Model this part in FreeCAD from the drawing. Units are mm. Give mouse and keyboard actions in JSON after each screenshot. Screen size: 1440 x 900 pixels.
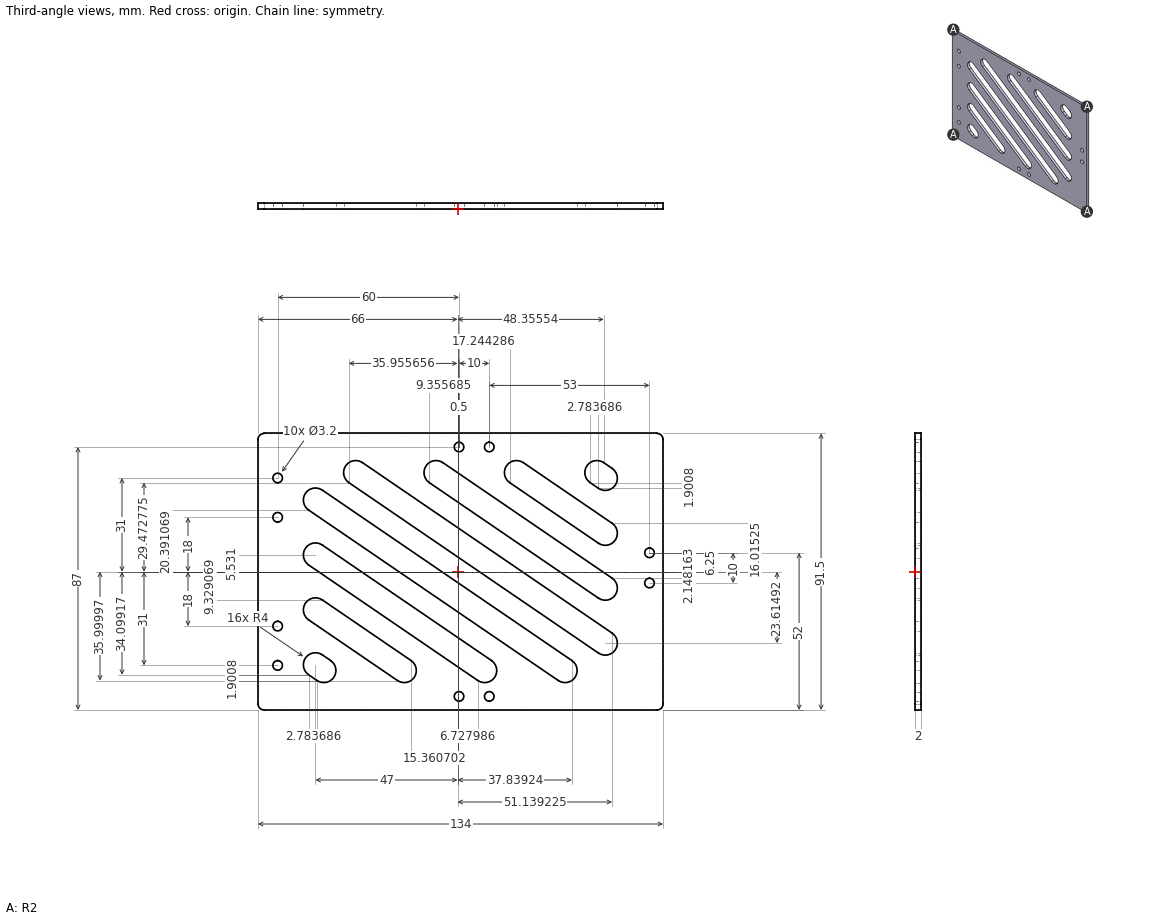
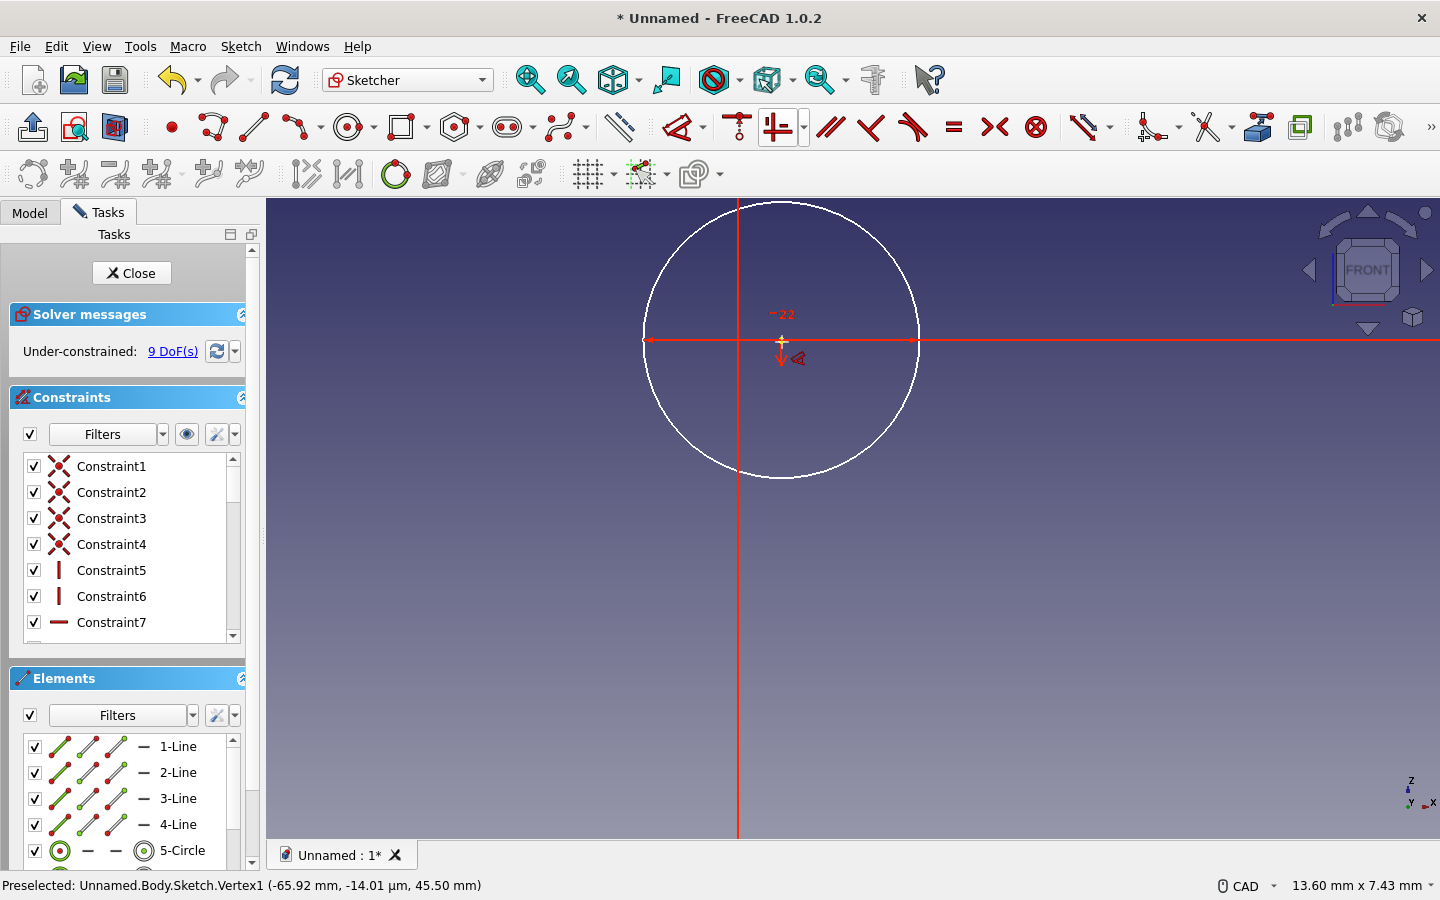
{"action": "left_click", "coordinate": [781, 340]}
{"action": "left_click", "coordinate": [760, 306]}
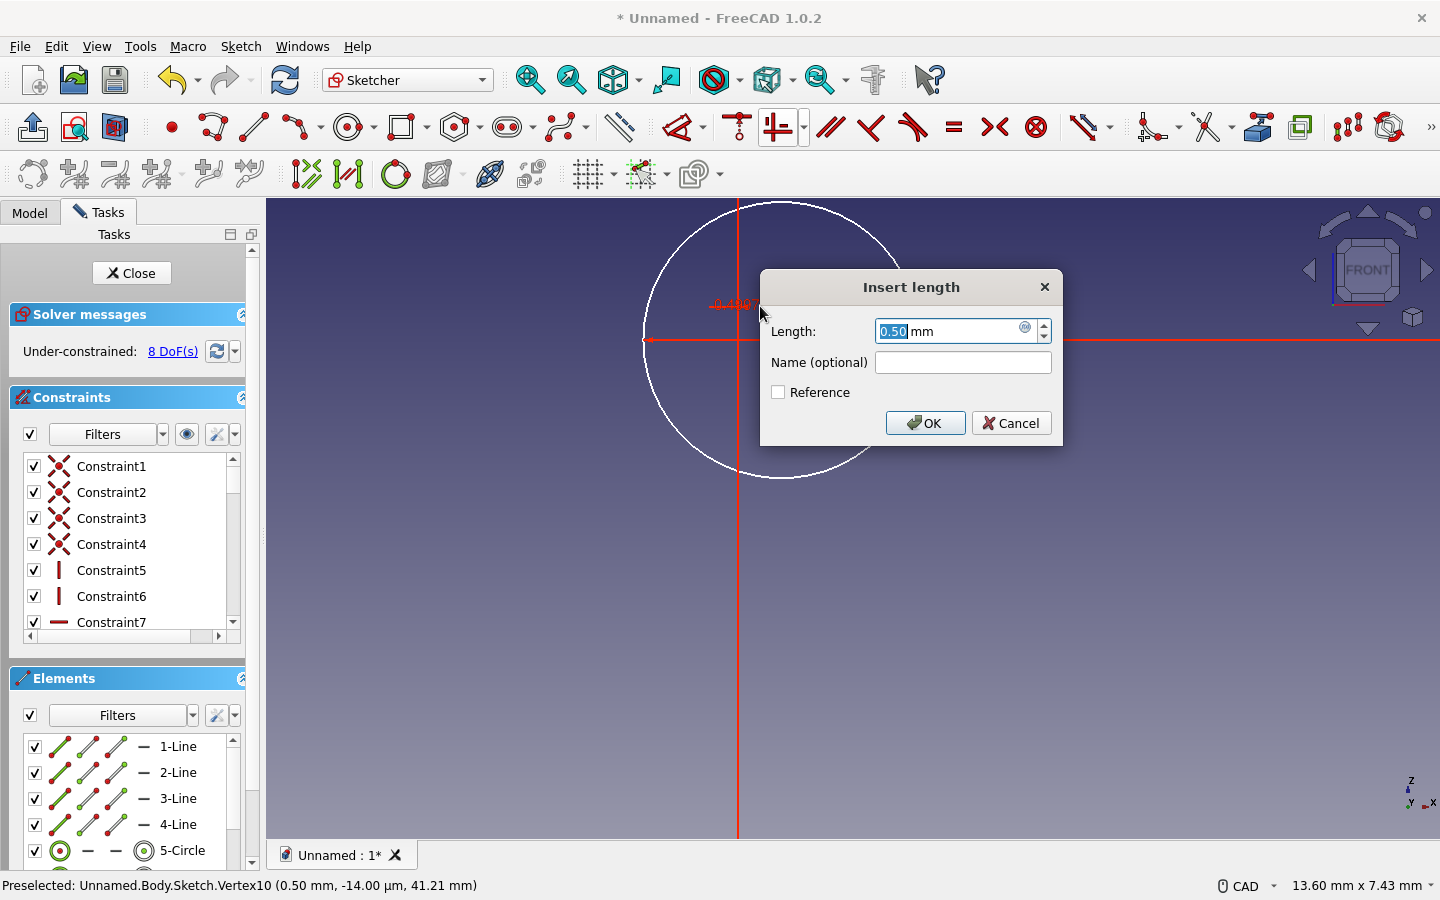
{"action": "type", "text": "0.5"}
{"action": "key", "text": "Return"}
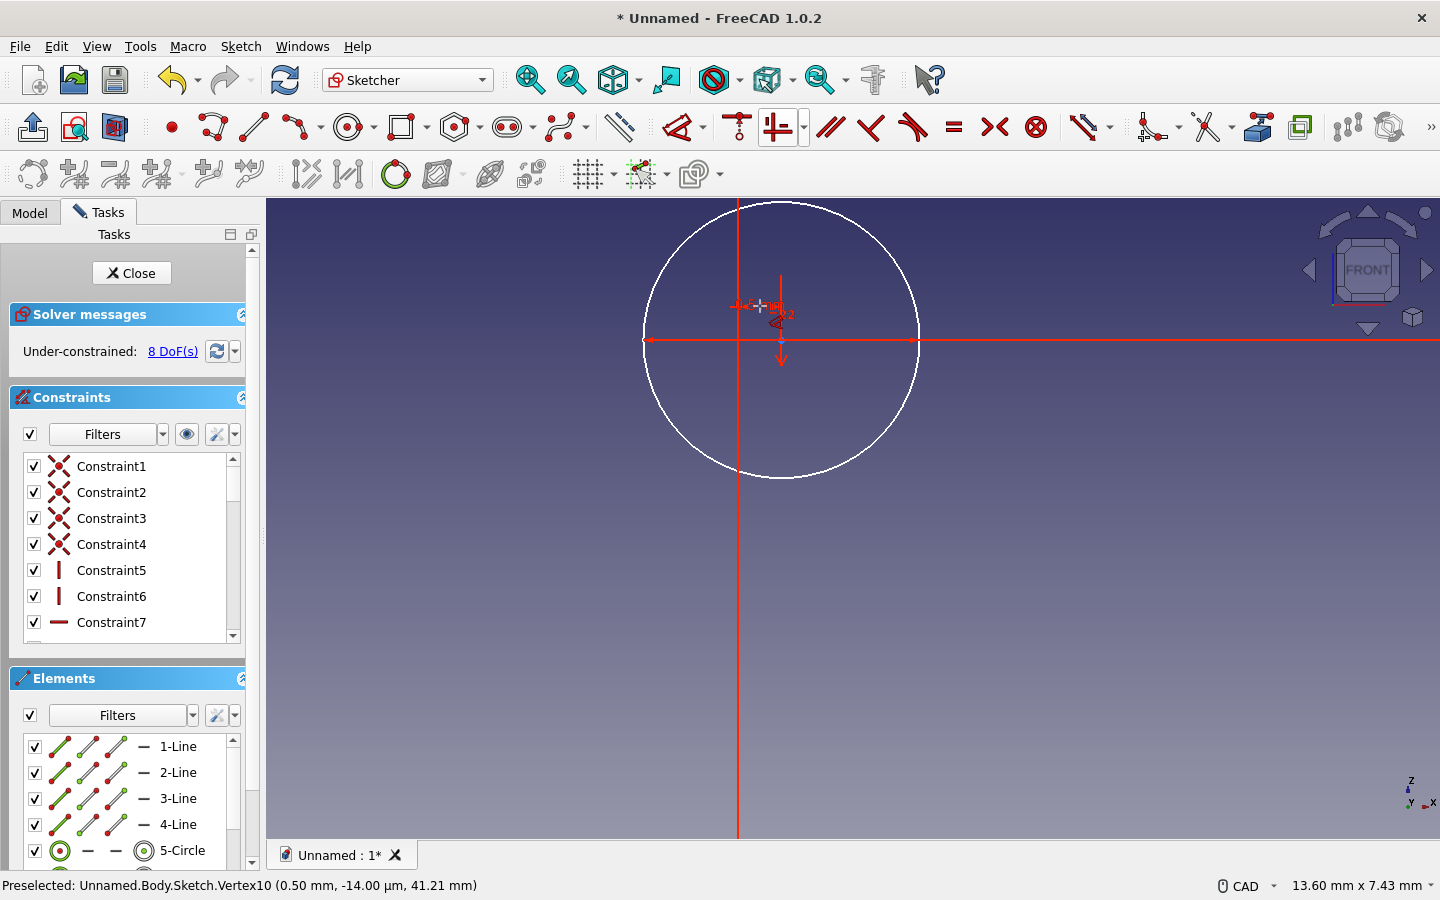
{"action": "scroll", "coordinate": [782, 341], "scroll_direction": "down", "scroll_amount": 15}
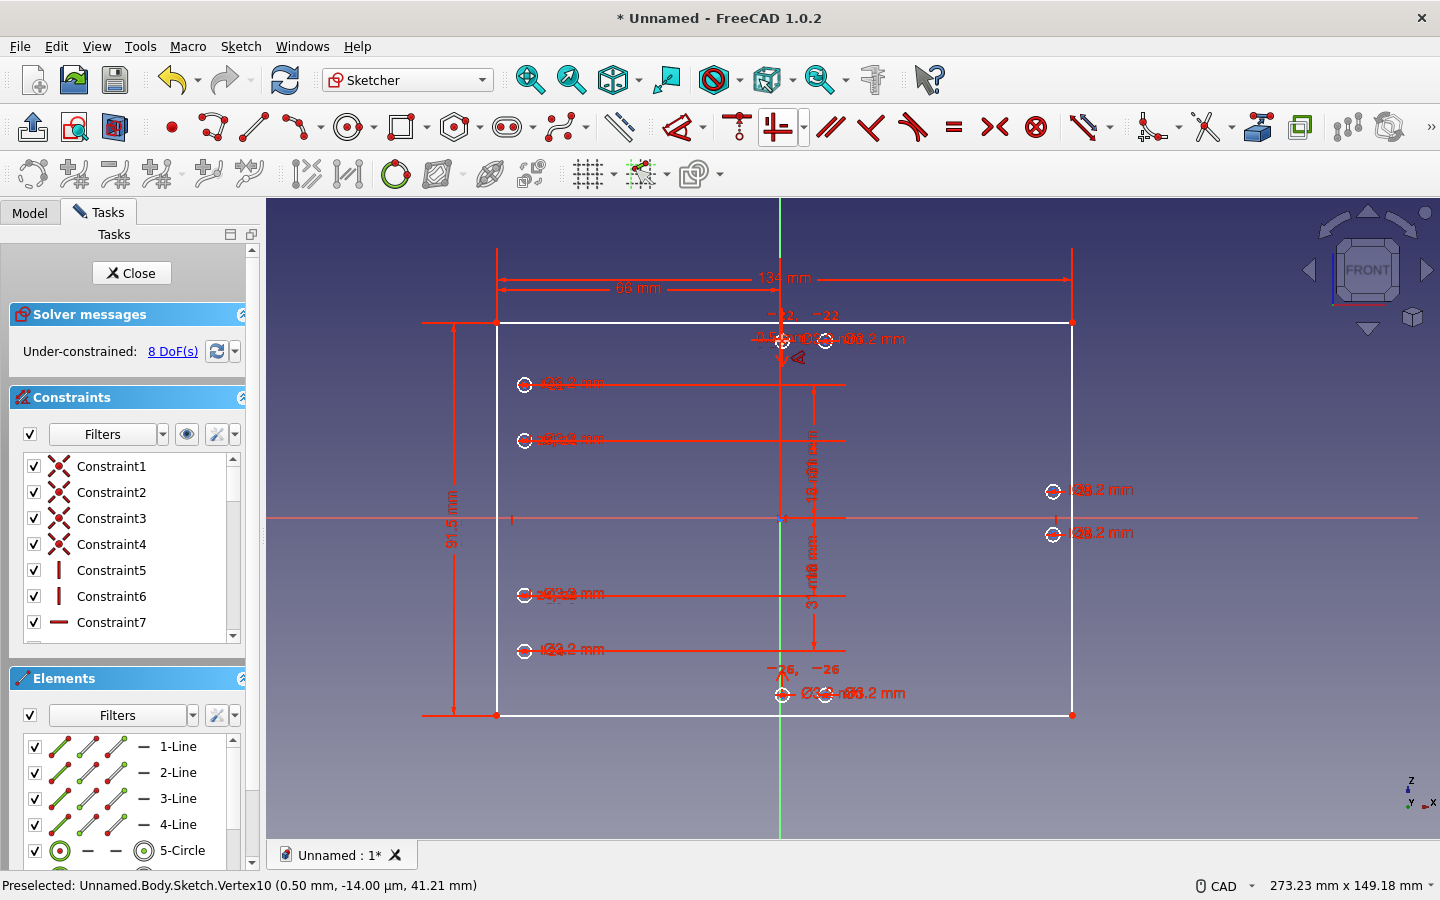
{"action": "left_click", "coordinate": [525, 385]}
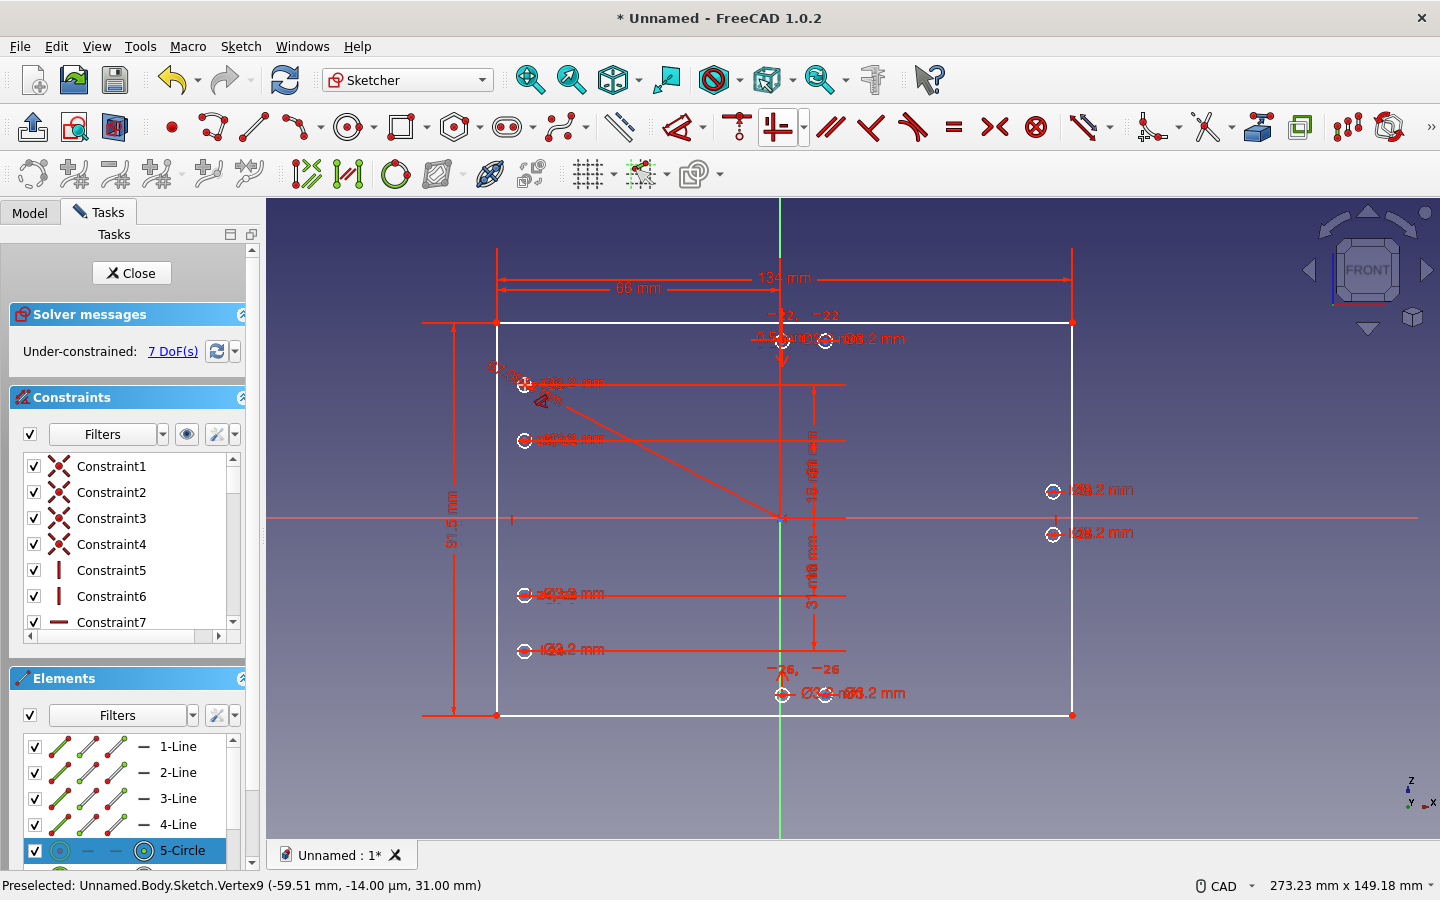
{"action": "left_click", "coordinate": [782, 341]}
{"action": "left_click", "coordinate": [713, 307]}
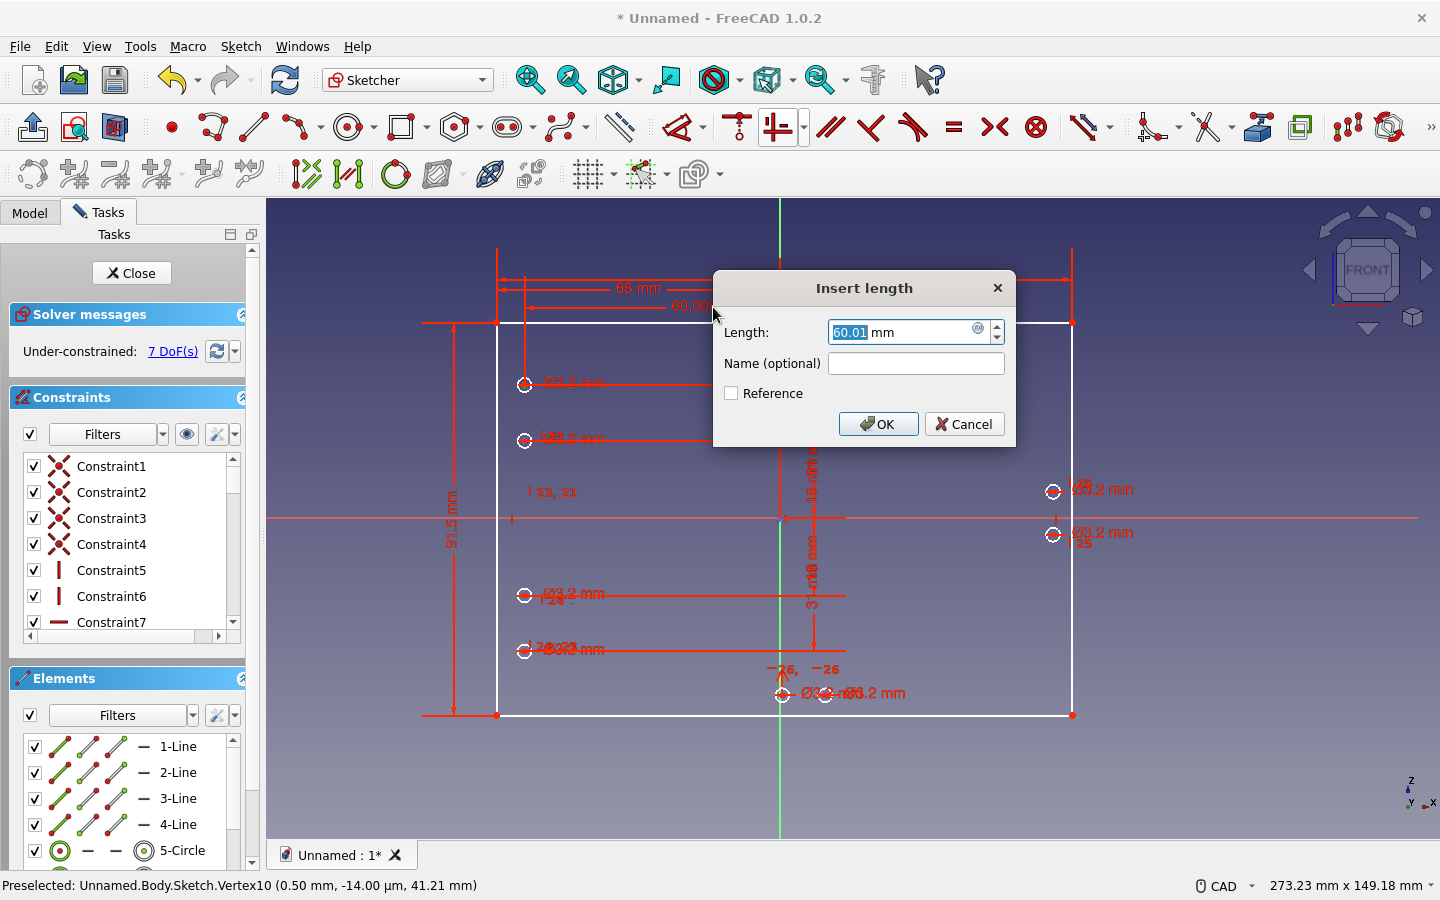
{"action": "type", "text": "60"}
{"action": "key", "text": "Return"}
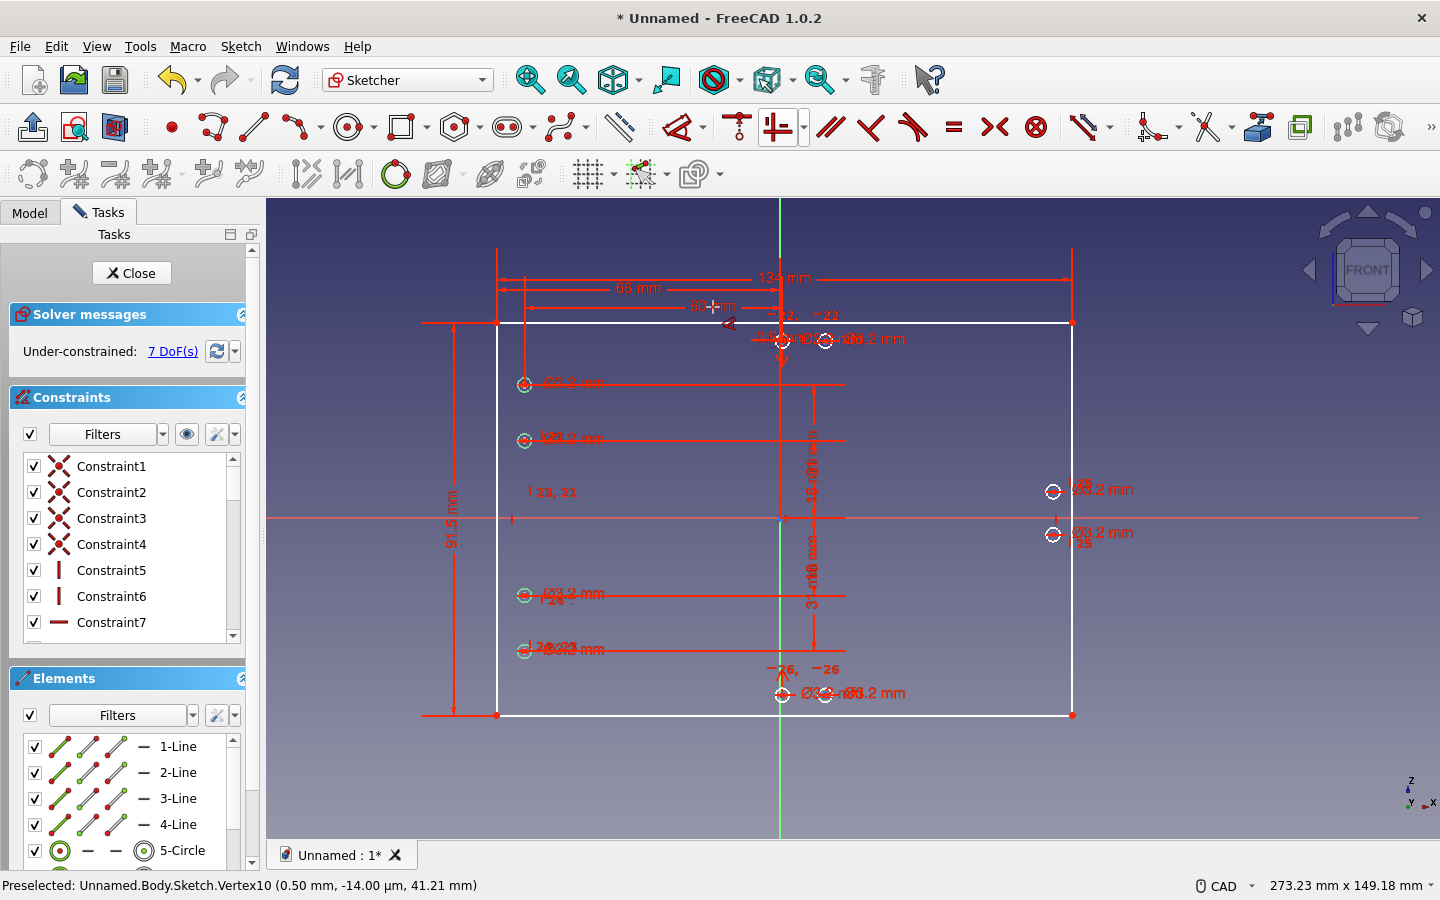
{"action": "left_click", "coordinate": [497, 716]}